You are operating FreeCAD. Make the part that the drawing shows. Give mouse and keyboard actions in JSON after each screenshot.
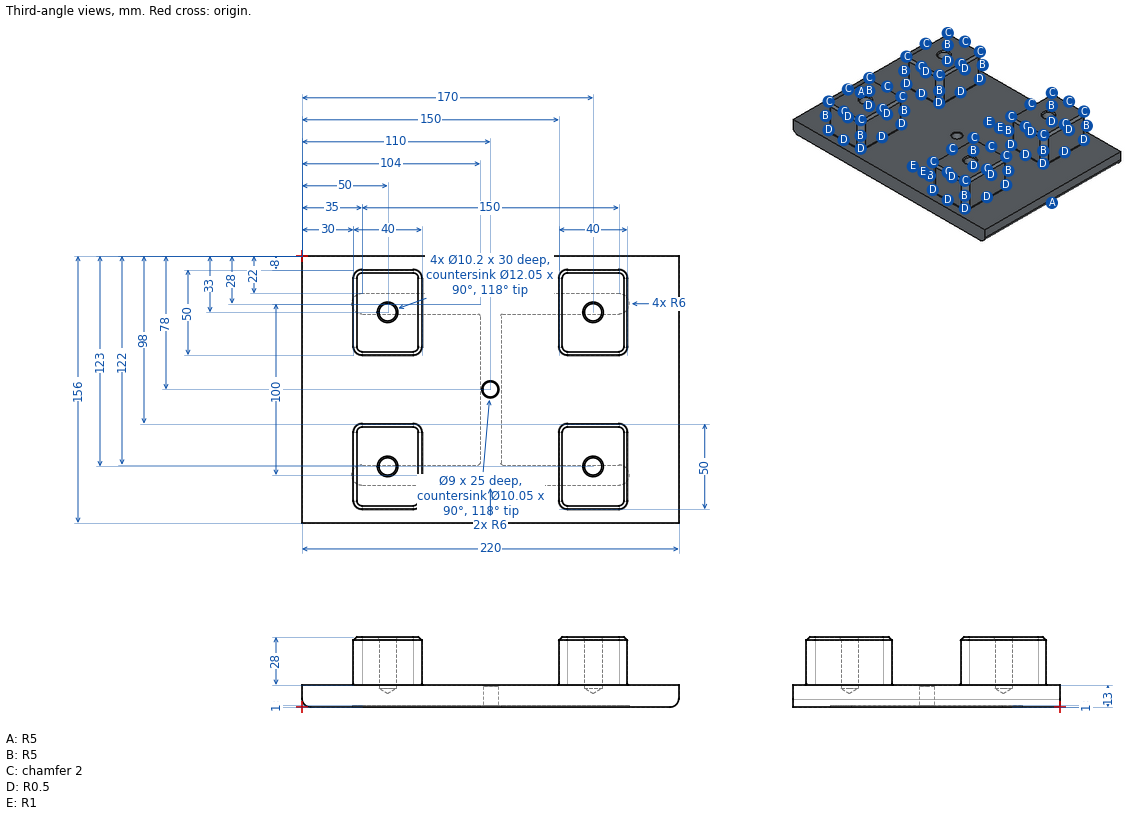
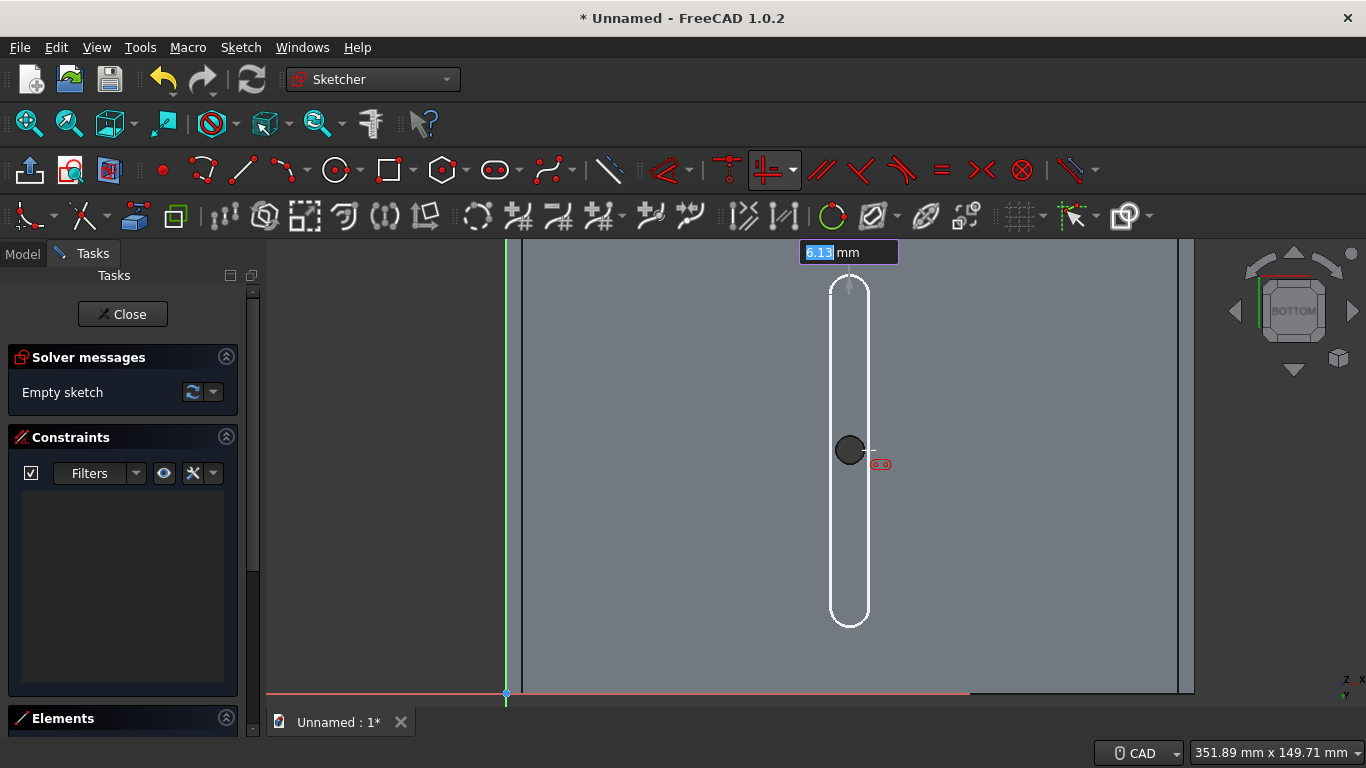
{"action": "left_click", "coordinate": [869, 450]}
{"action": "key", "text": "Escape"}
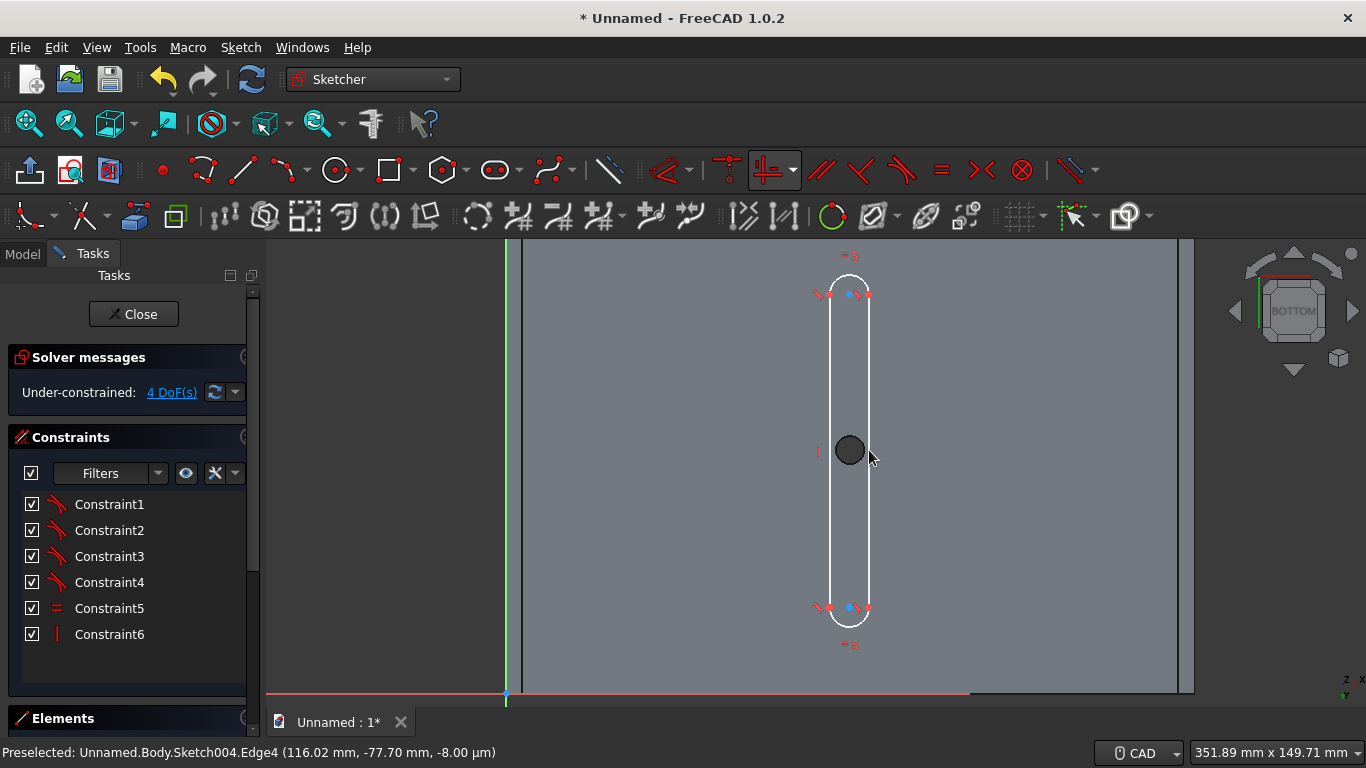
{"action": "key", "text": "d"}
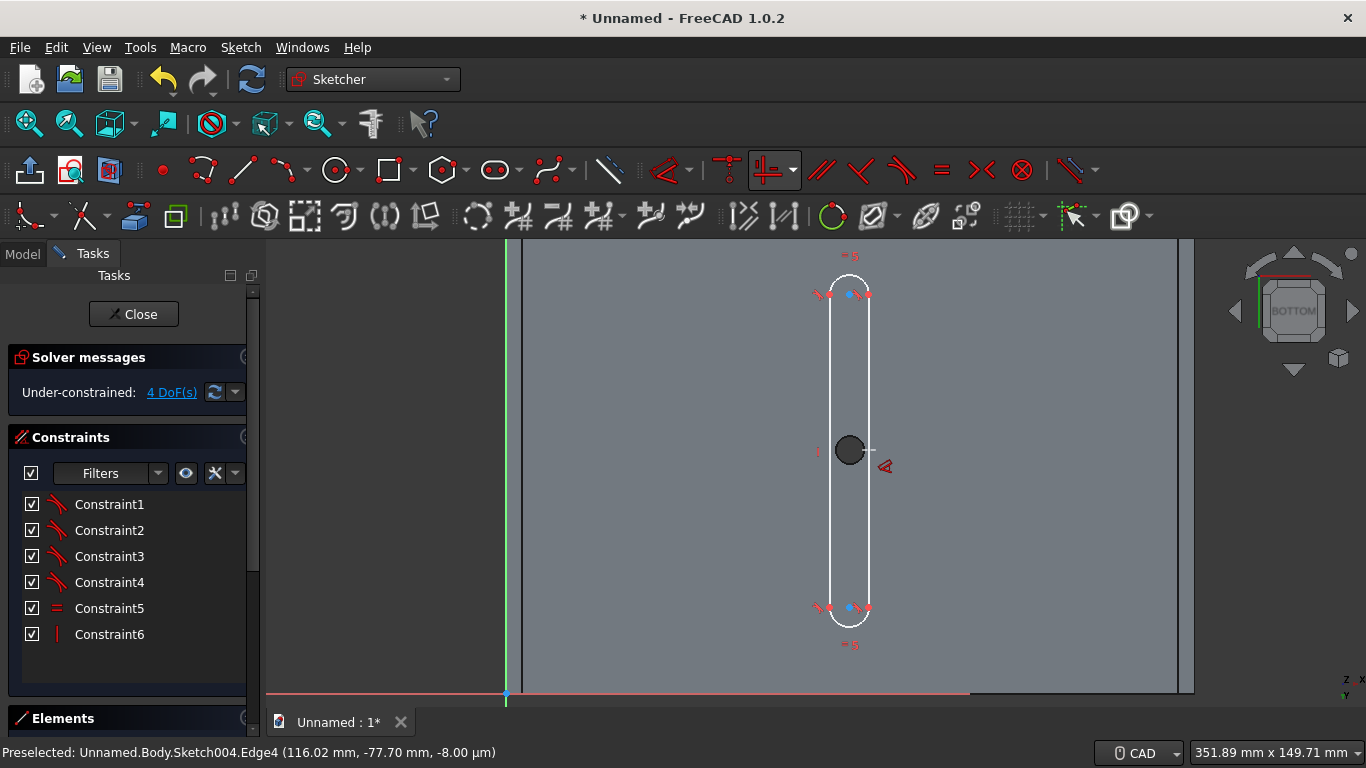
{"action": "scroll", "coordinate": [838, 623], "scroll_direction": "up", "scroll_amount": 4}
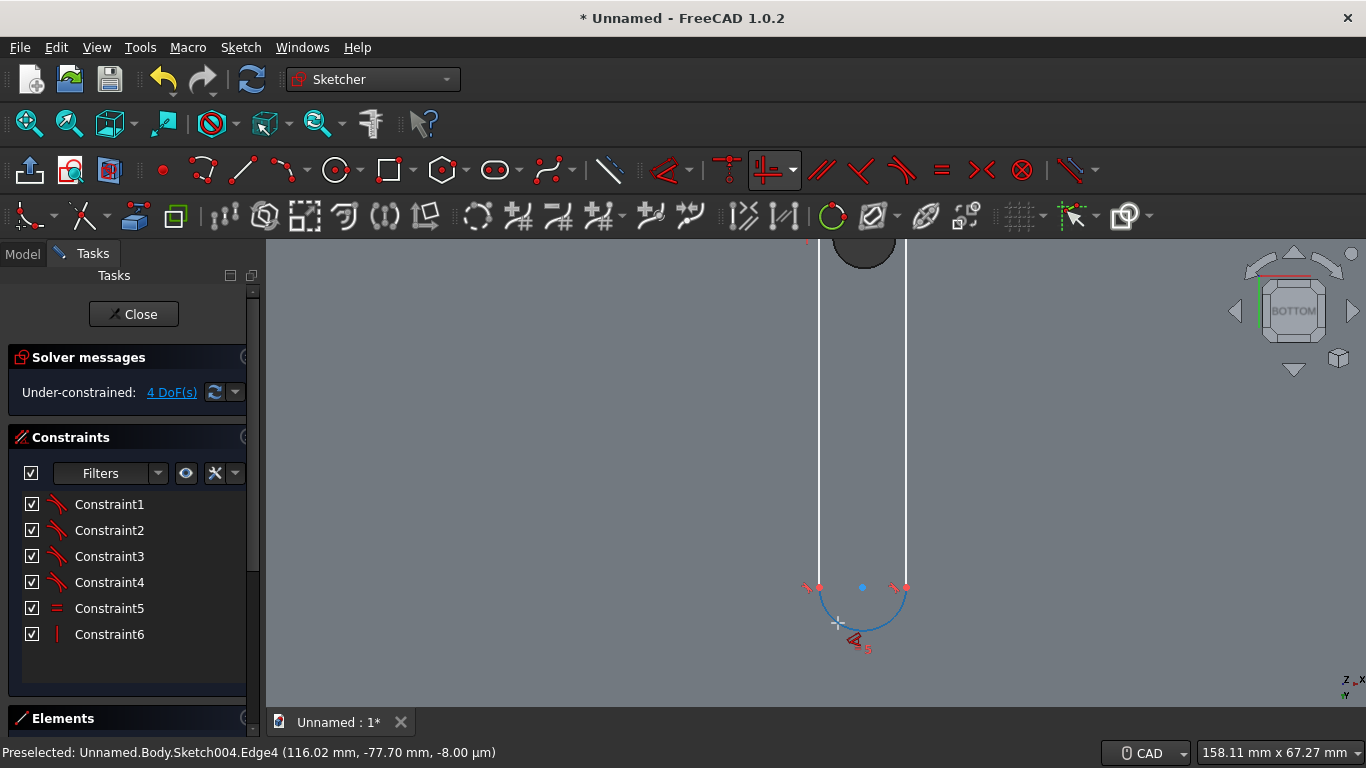
{"action": "left_click", "coordinate": [837, 622]}
{"action": "left_click", "coordinate": [818, 648]}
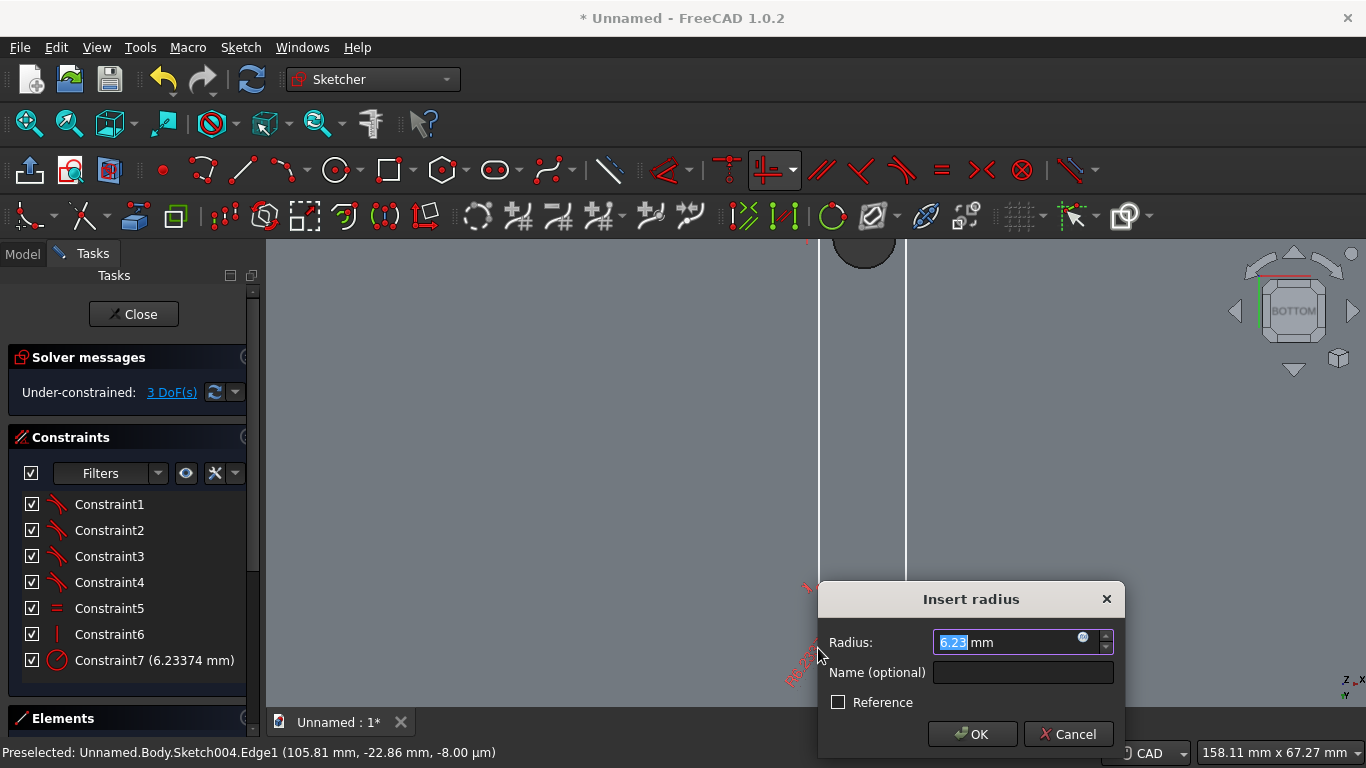
{"action": "type", "text": "6"}
{"action": "key", "text": "Return"}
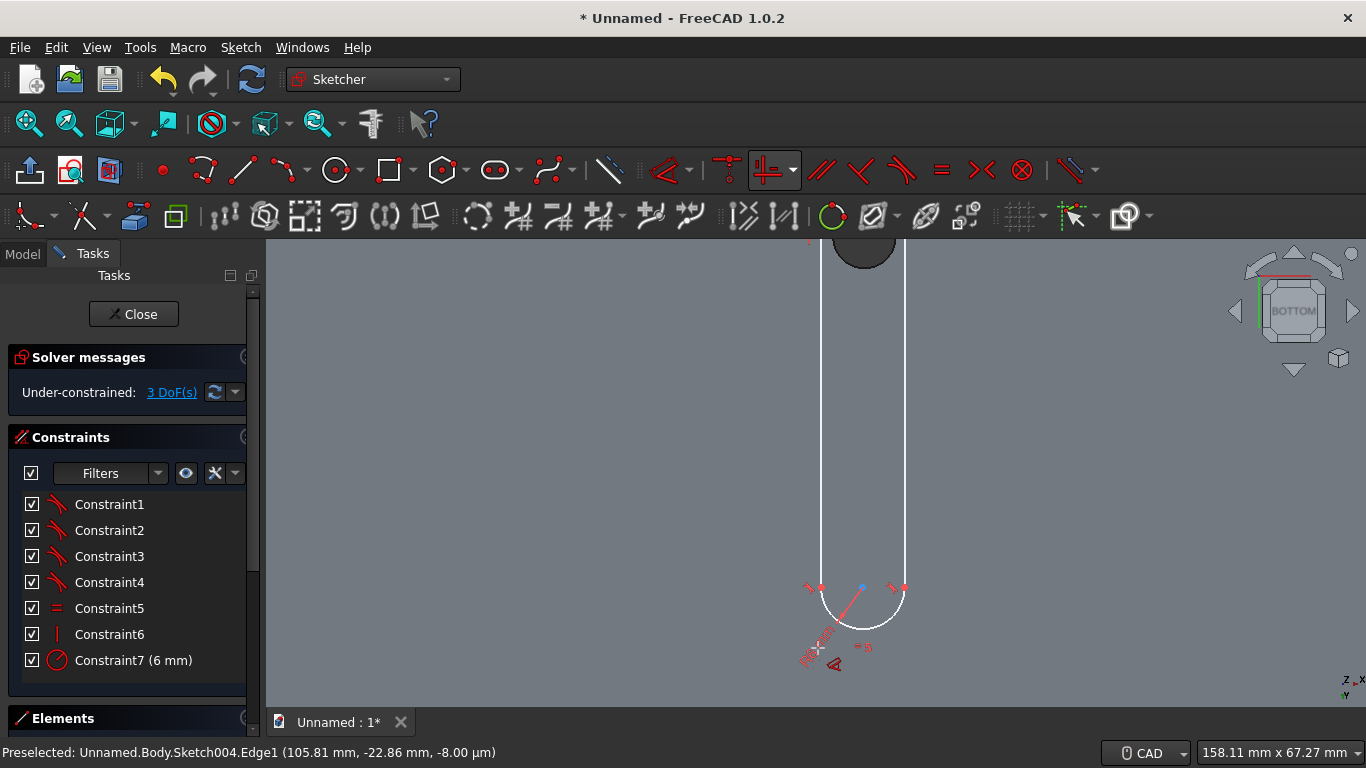
{"action": "scroll", "coordinate": [853, 542], "scroll_direction": "down", "scroll_amount": 6}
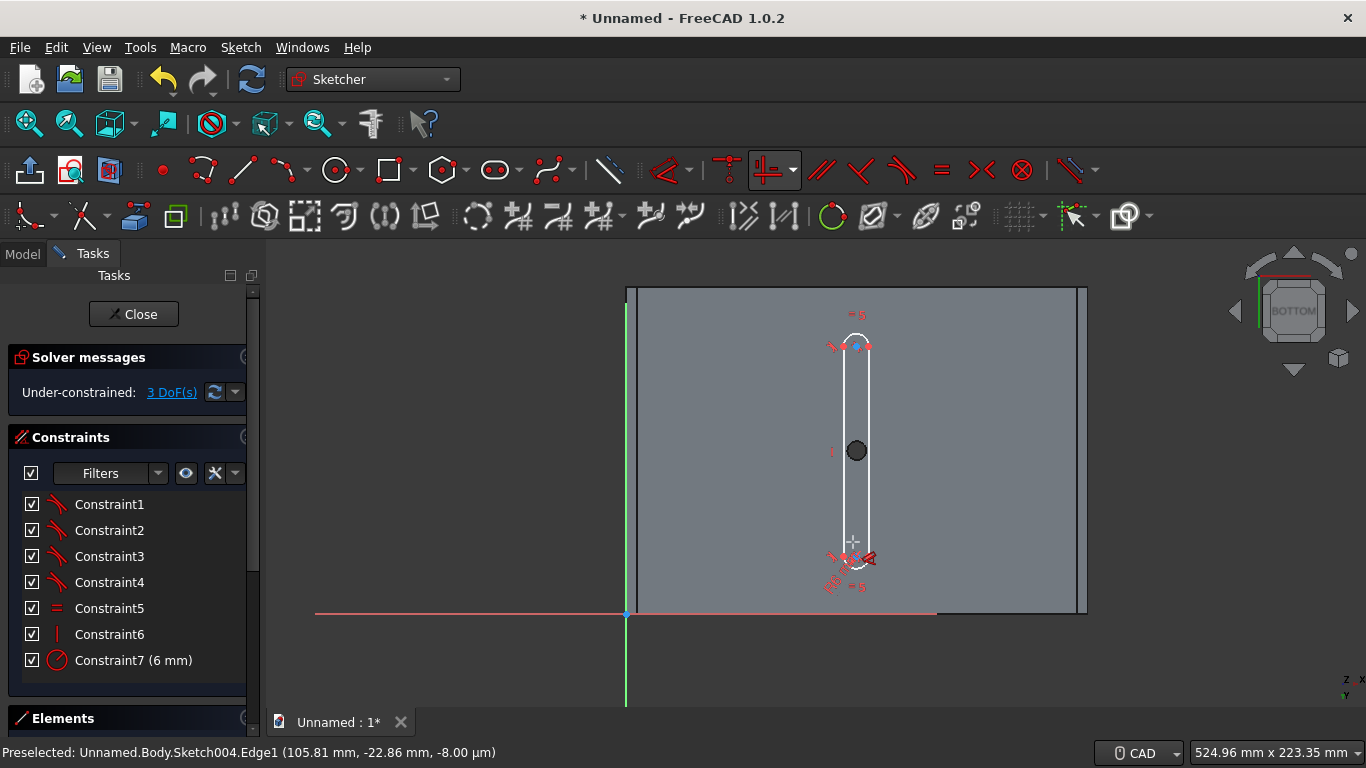
{"action": "left_click", "coordinate": [844, 493]}
{"action": "left_click", "coordinate": [810, 451]}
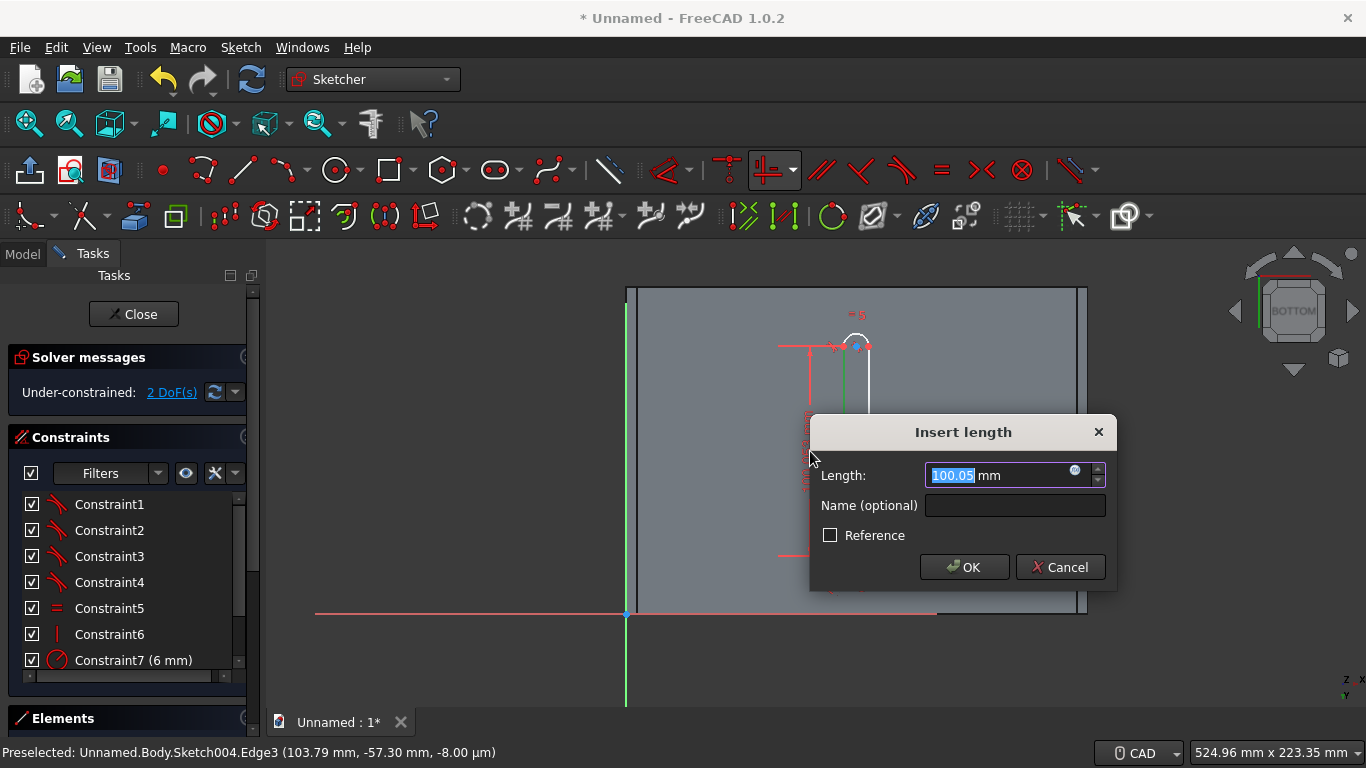
{"action": "type", "text": "100"}
{"action": "key", "text": "Return"}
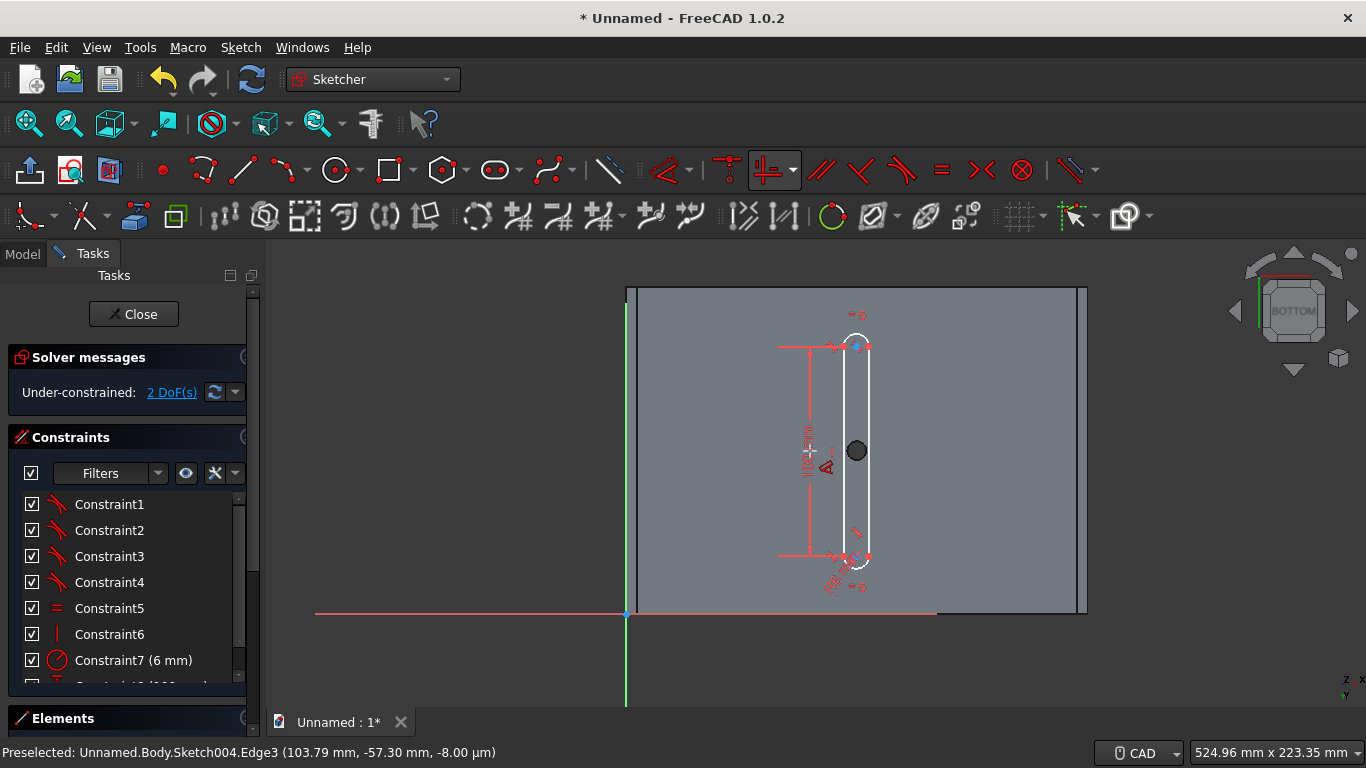
{"action": "left_click", "coordinate": [844, 556]}
{"action": "left_click", "coordinate": [592, 585]}